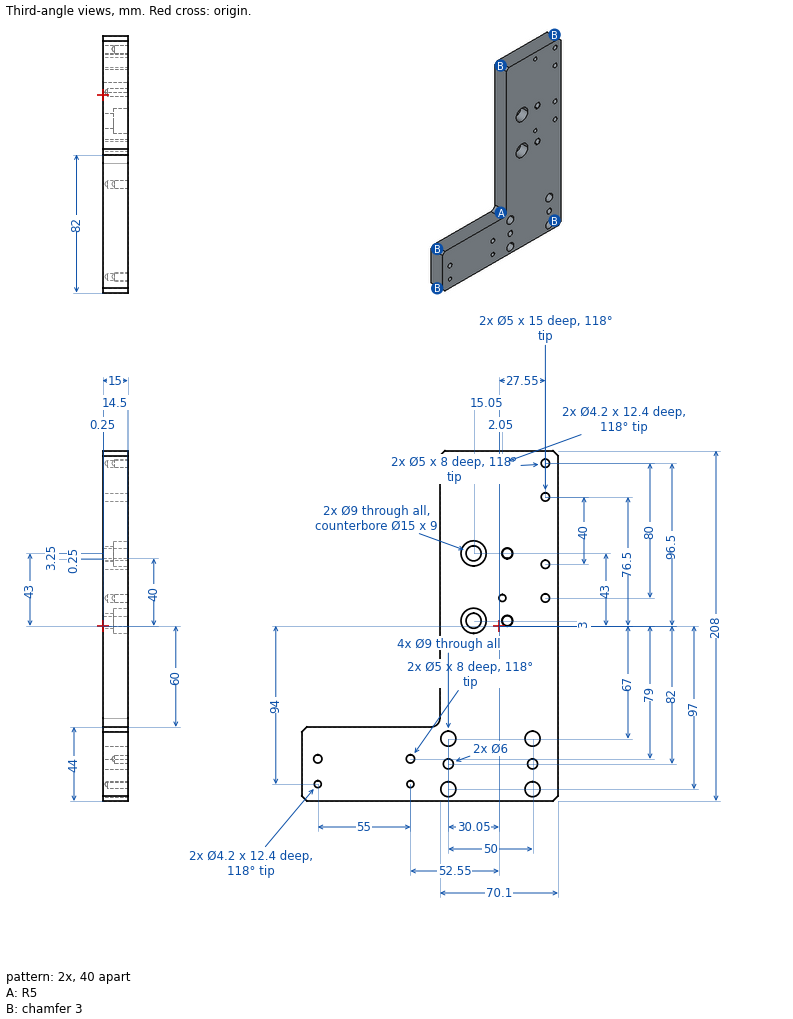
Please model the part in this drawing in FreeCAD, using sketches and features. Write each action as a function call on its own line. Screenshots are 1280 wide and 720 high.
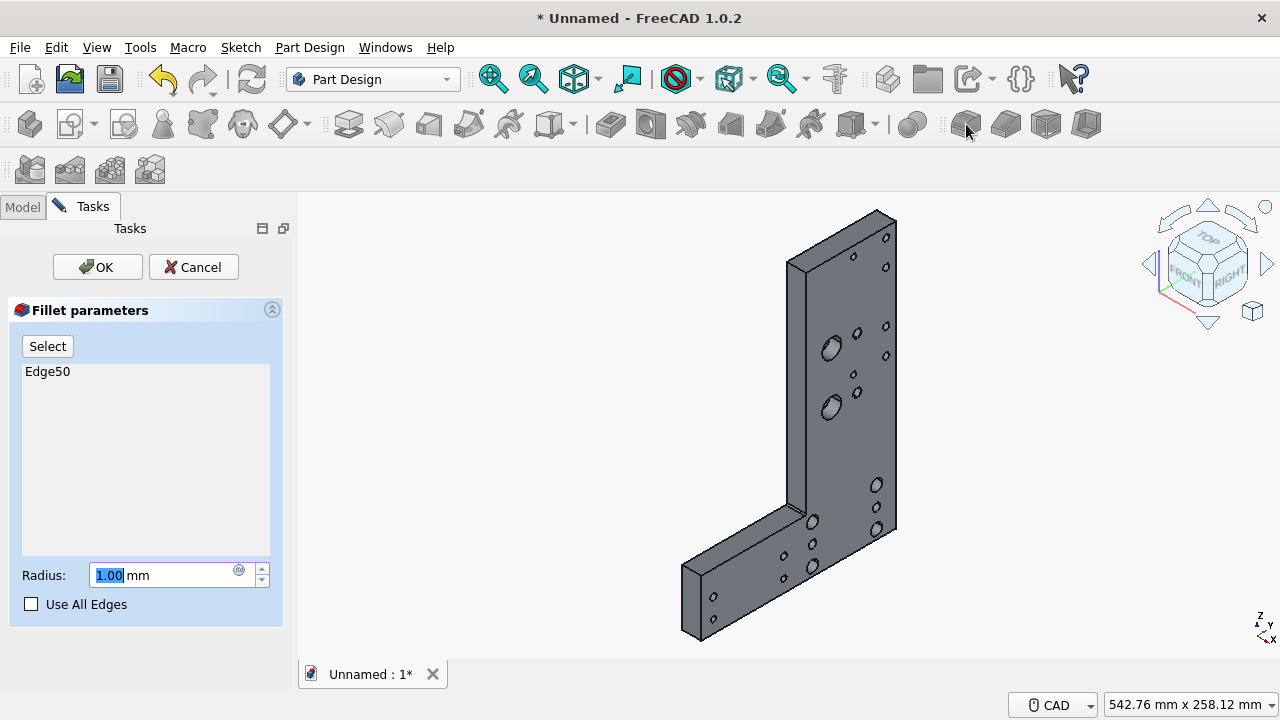
text(5)
key(Tab)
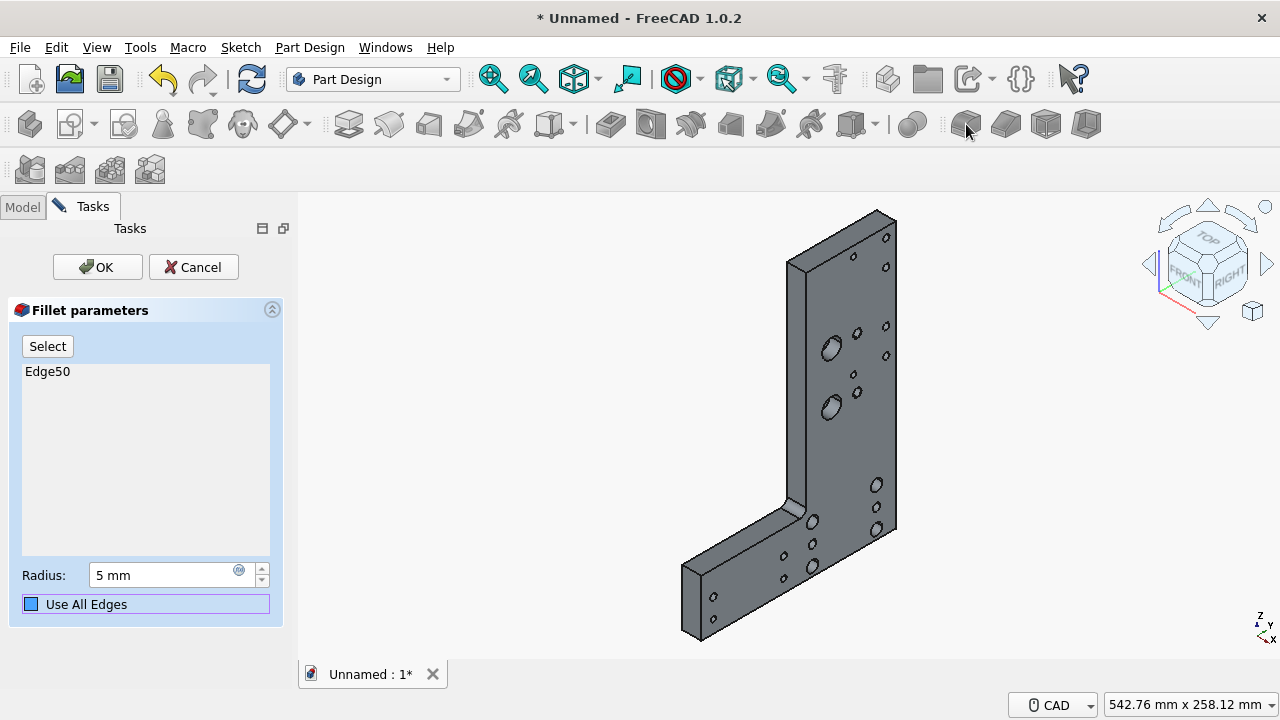
click(98, 267)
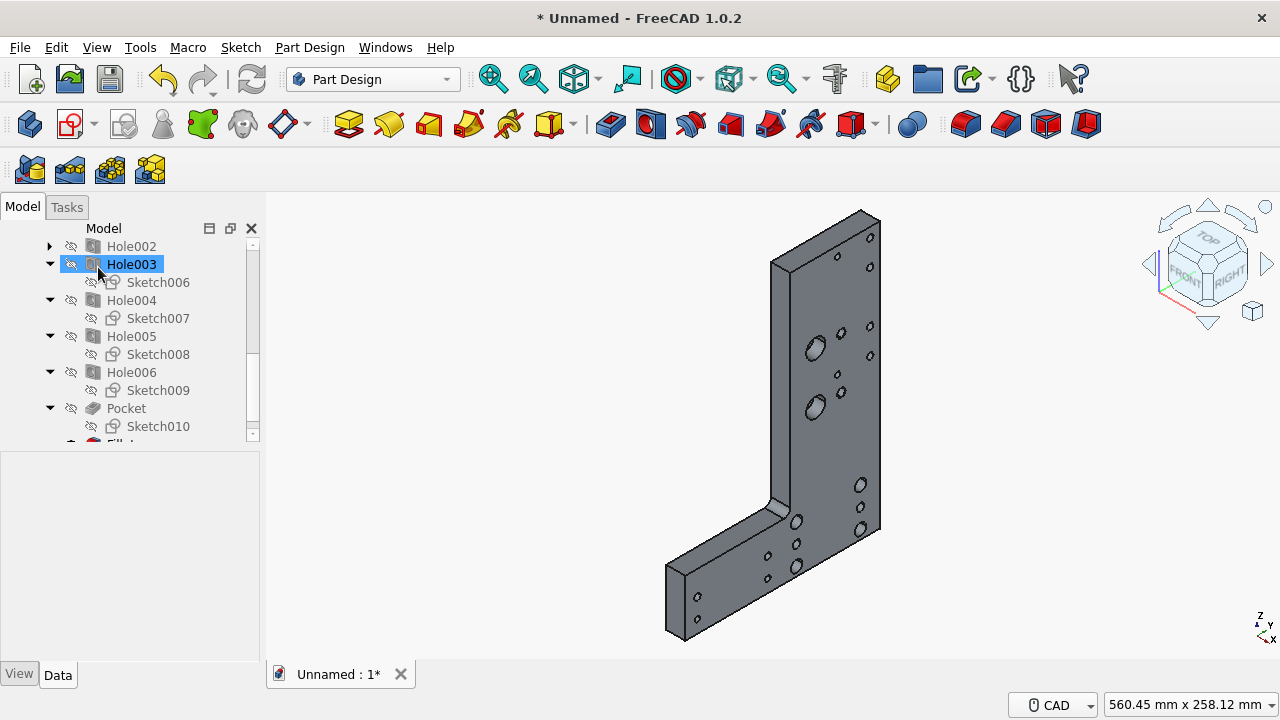
click(676, 569)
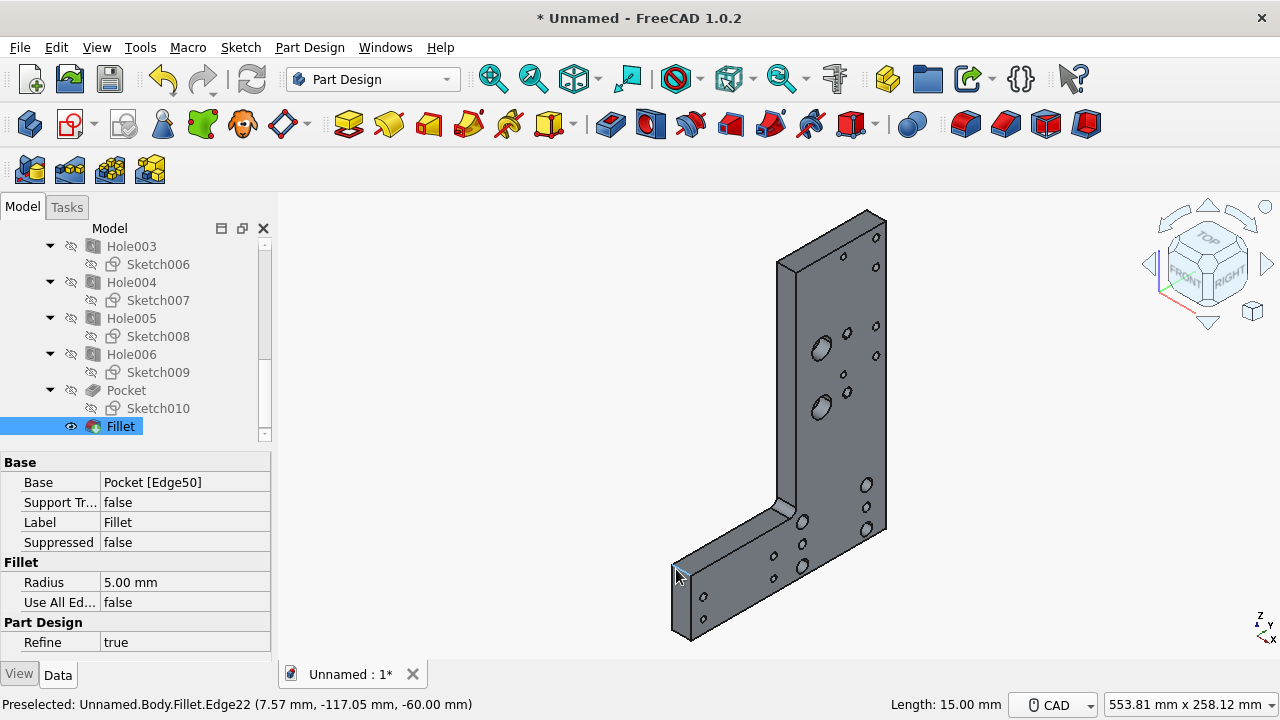
click(787, 266, ctrl)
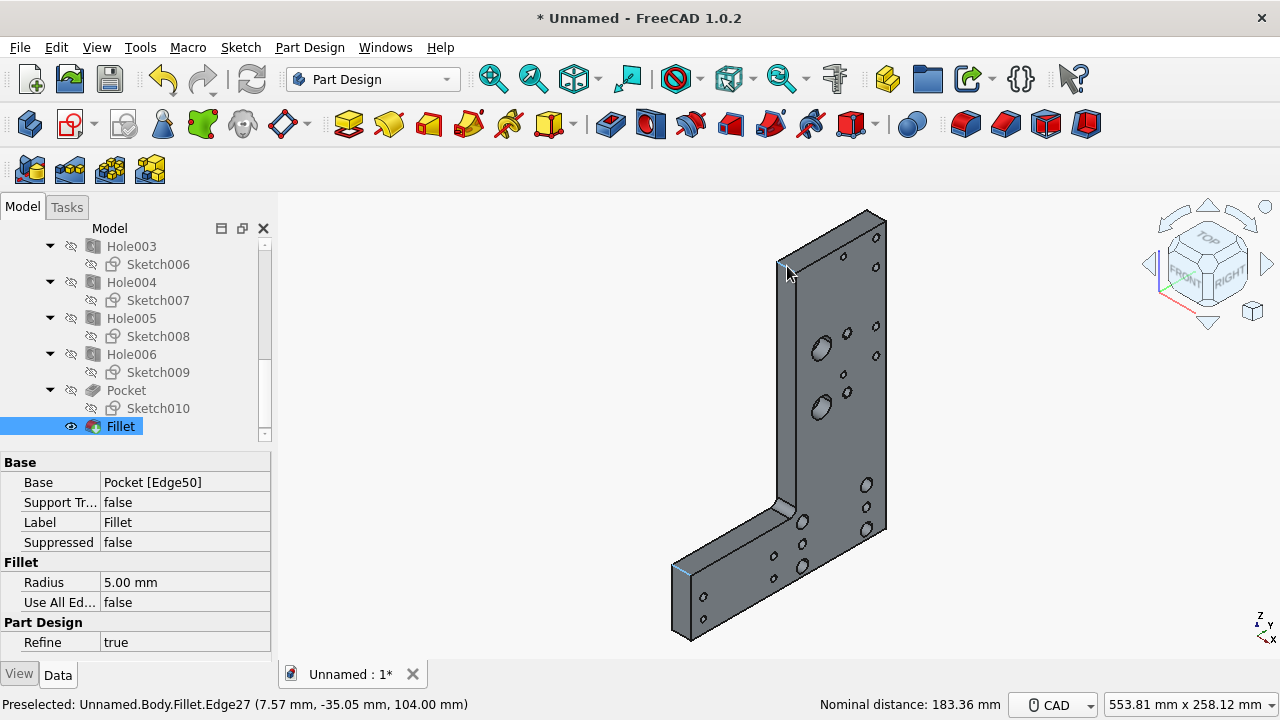
key(2)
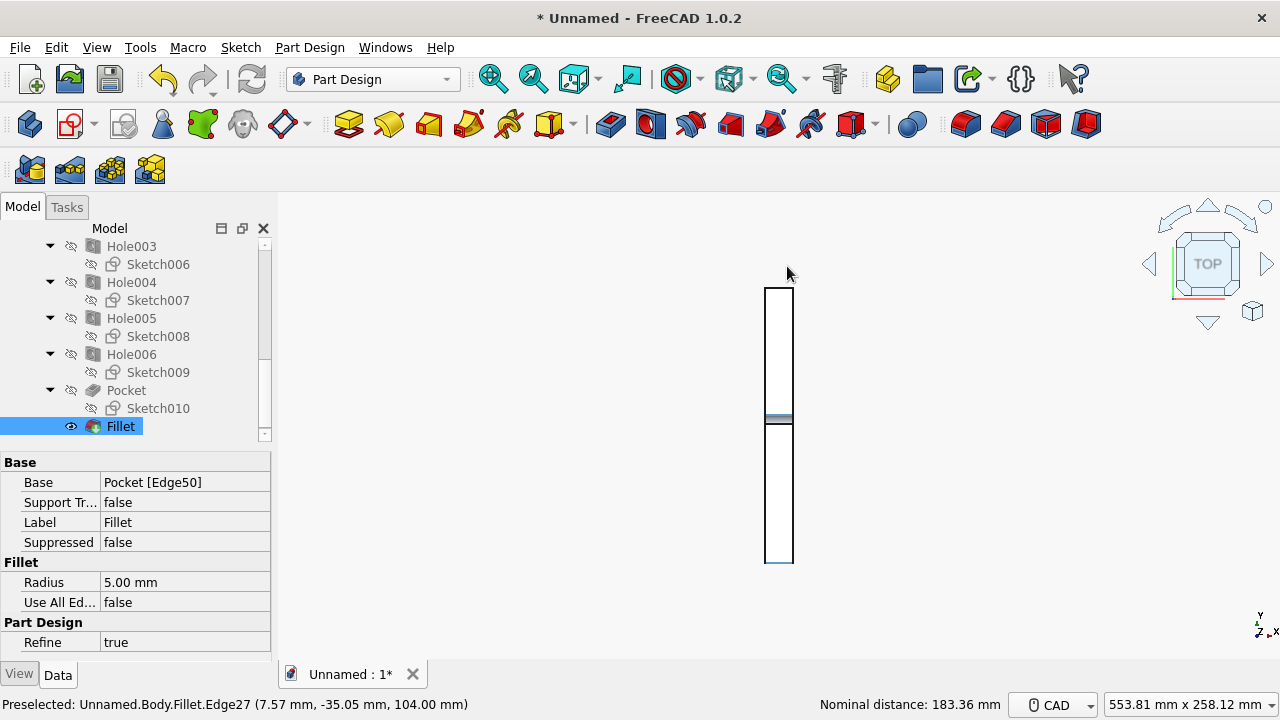
click(779, 287, ctrl)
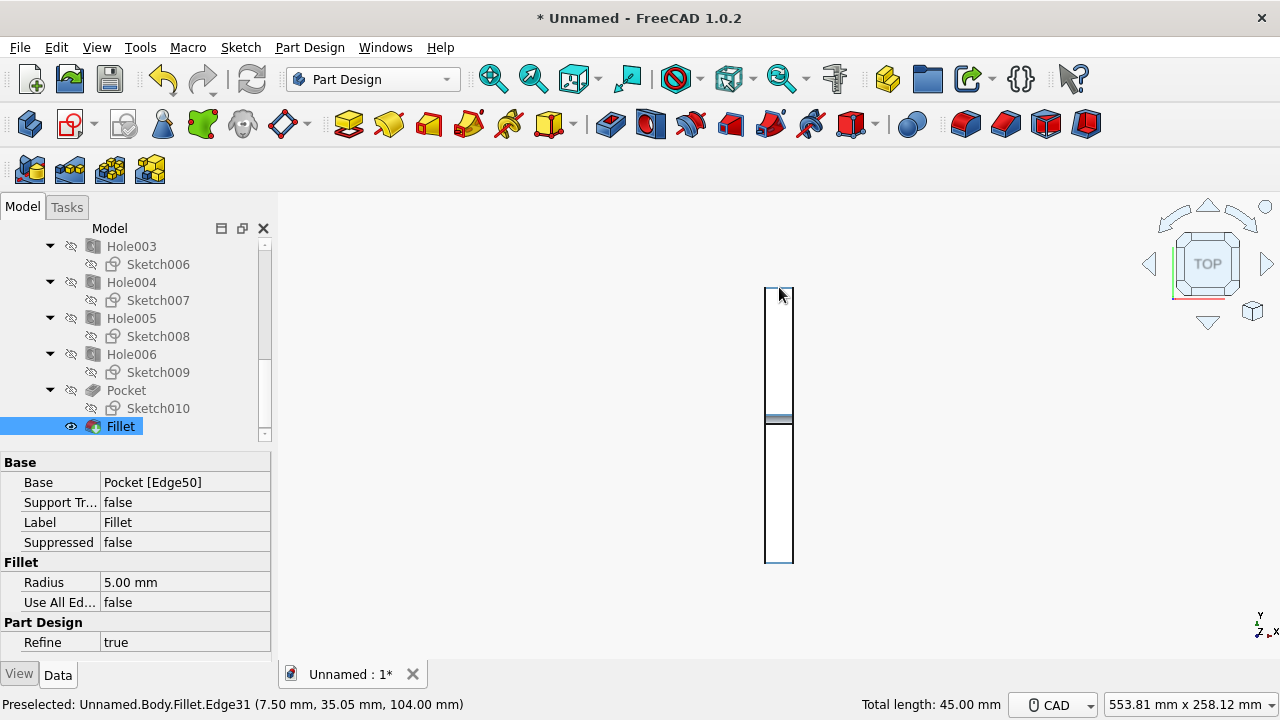
key(0)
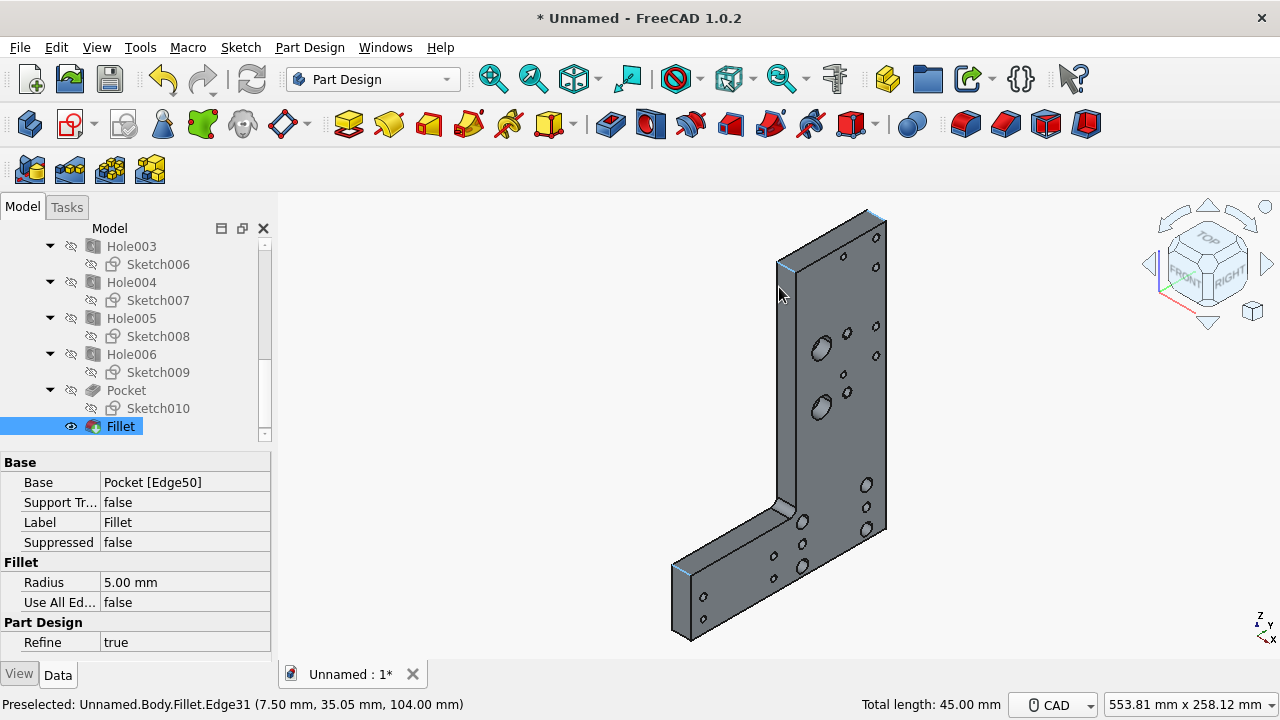
key(1)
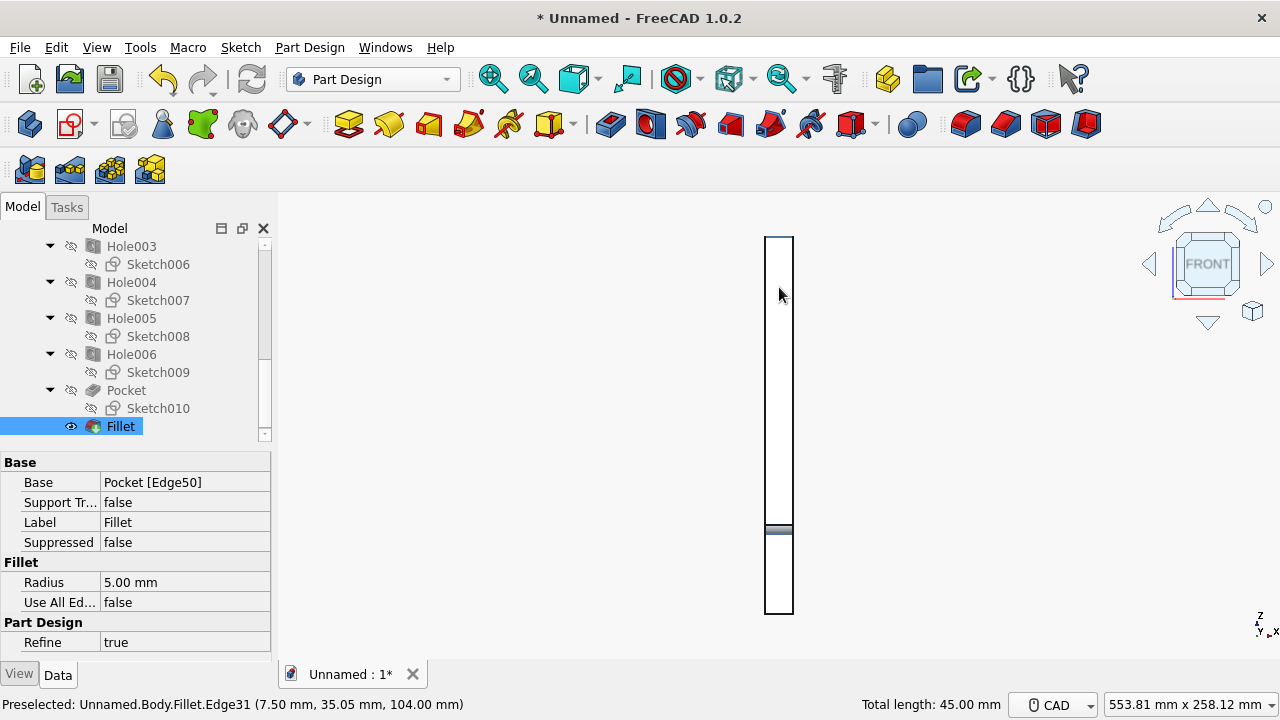
click(779, 613, ctrl)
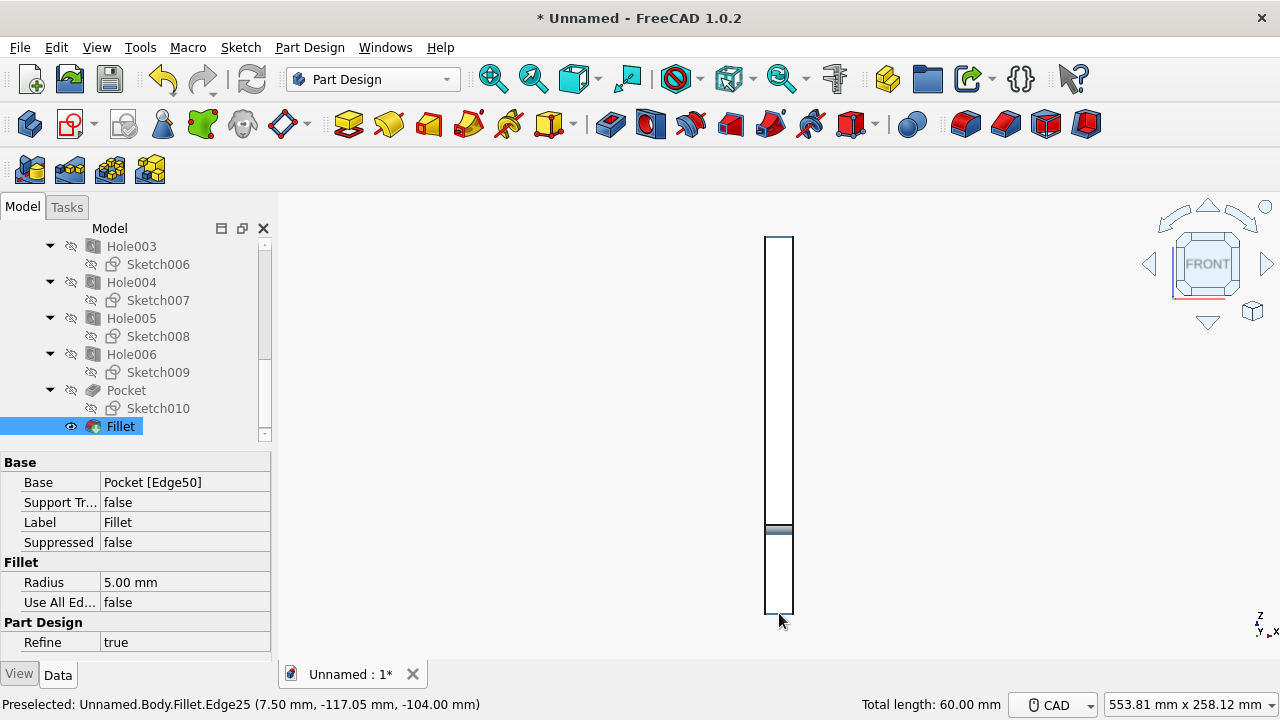
key(3)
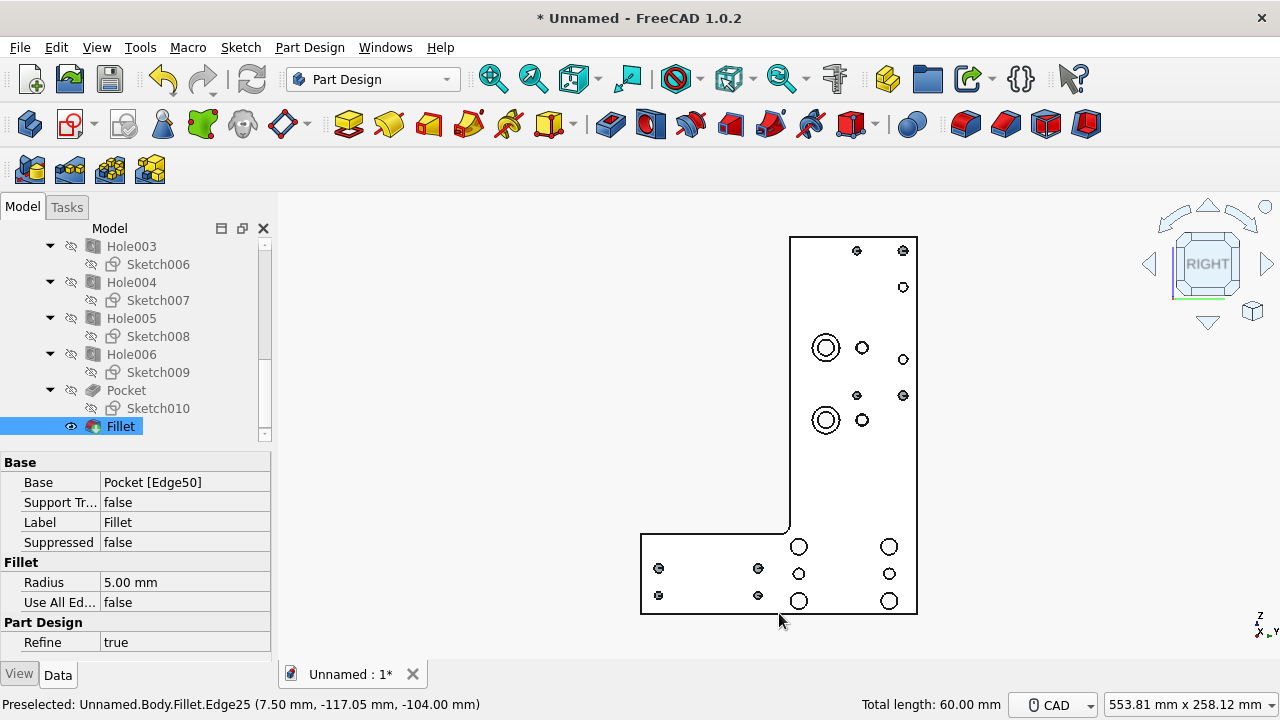
key(5)